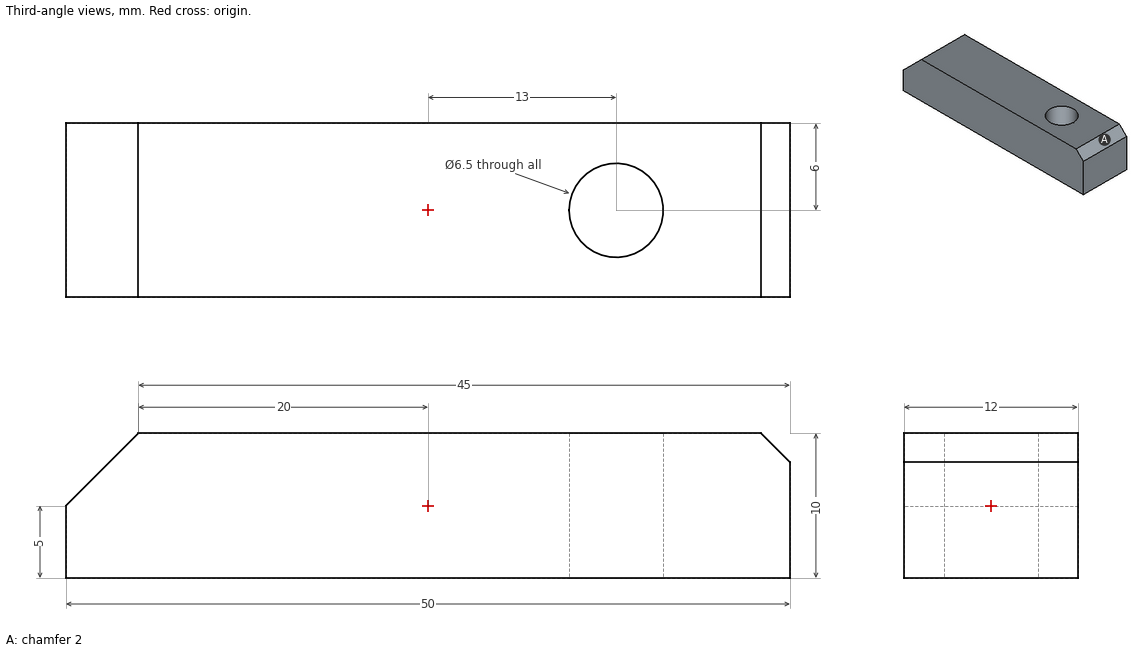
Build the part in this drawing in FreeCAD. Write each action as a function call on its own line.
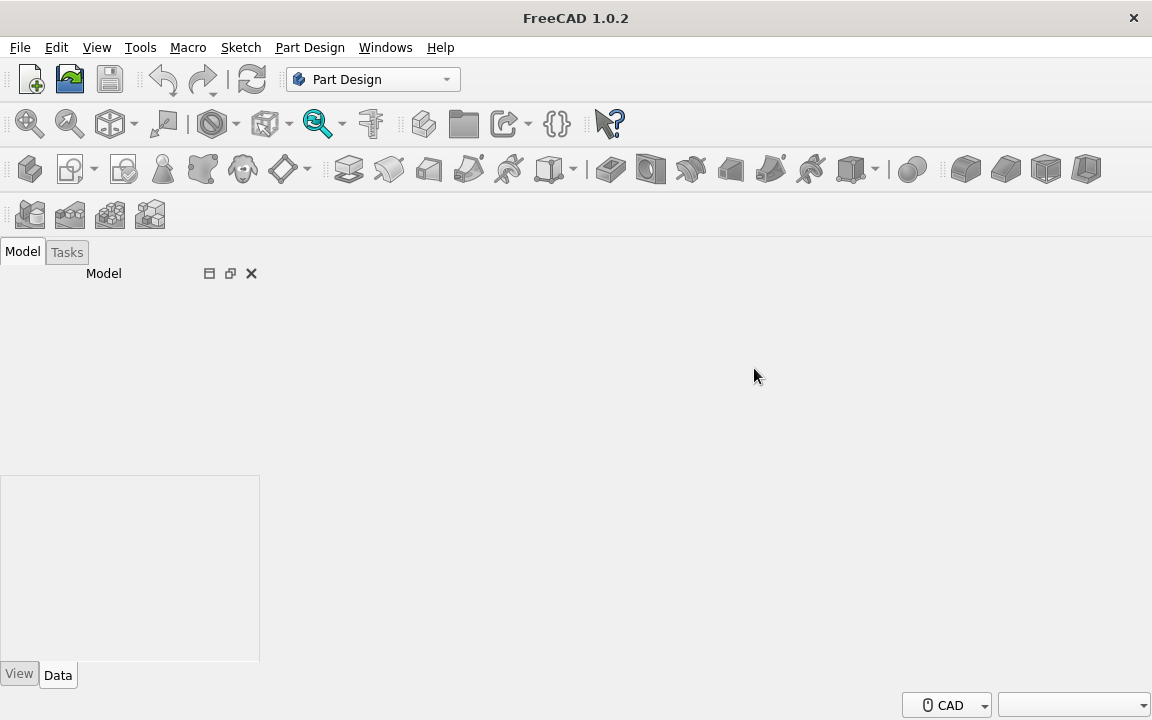
click(30, 80)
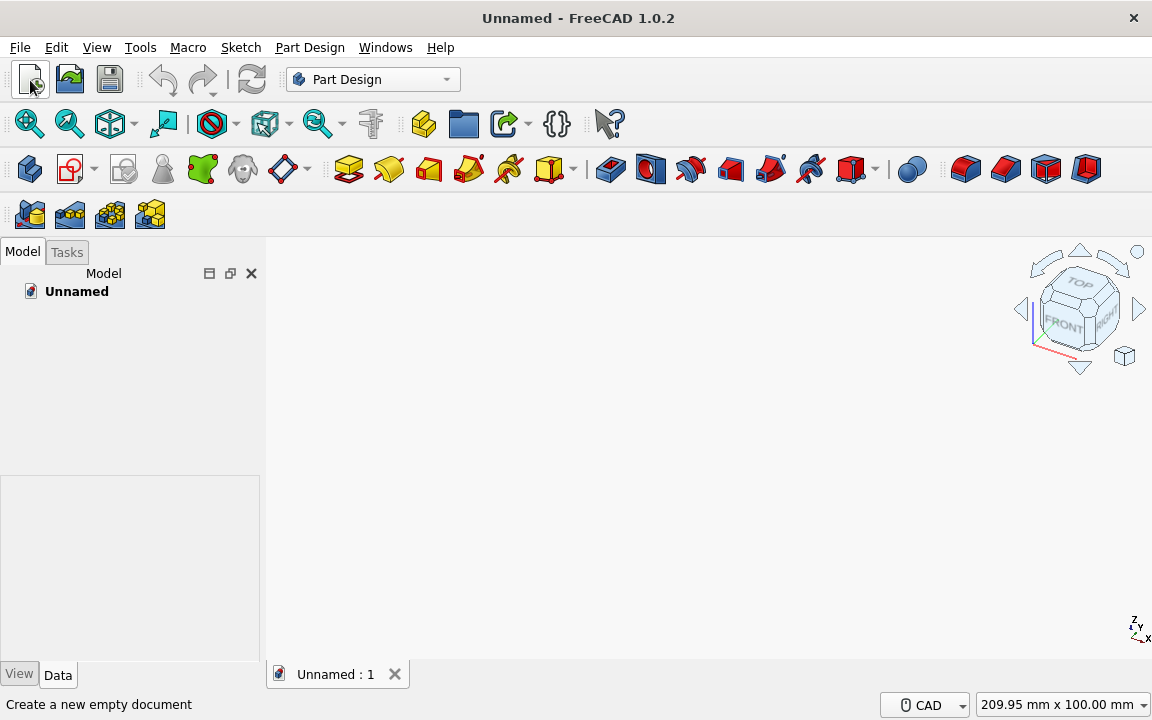
click(30, 170)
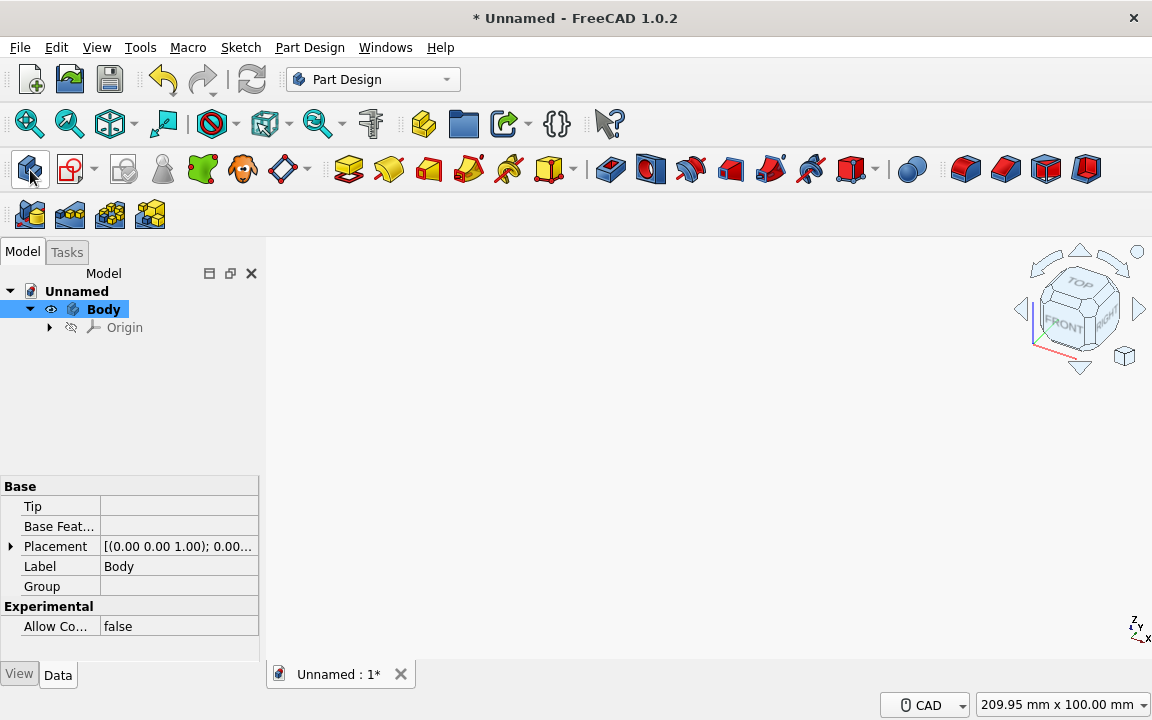
click(50, 327)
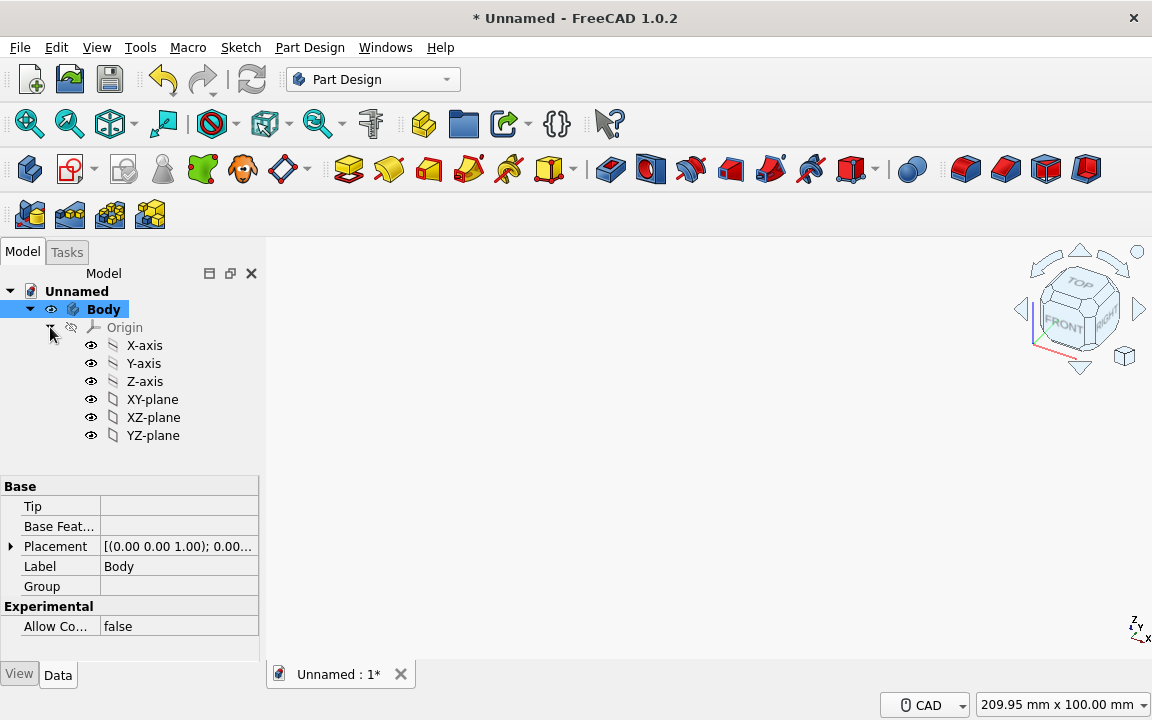
click(136, 417)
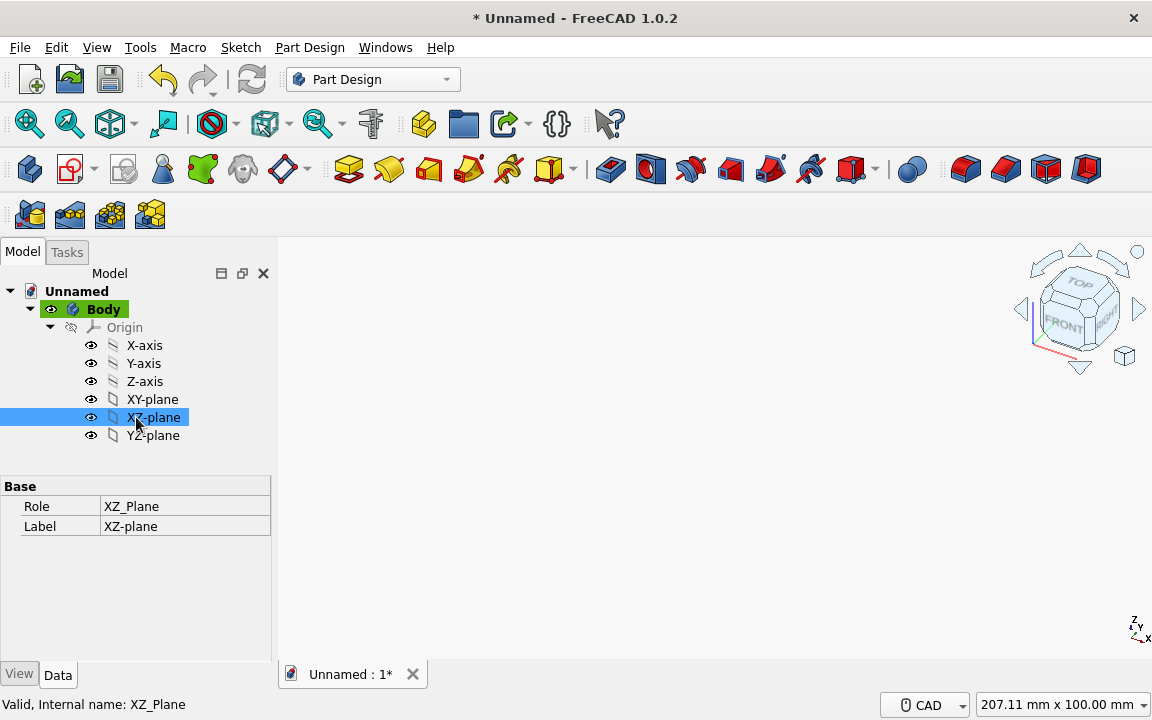
click(284, 170)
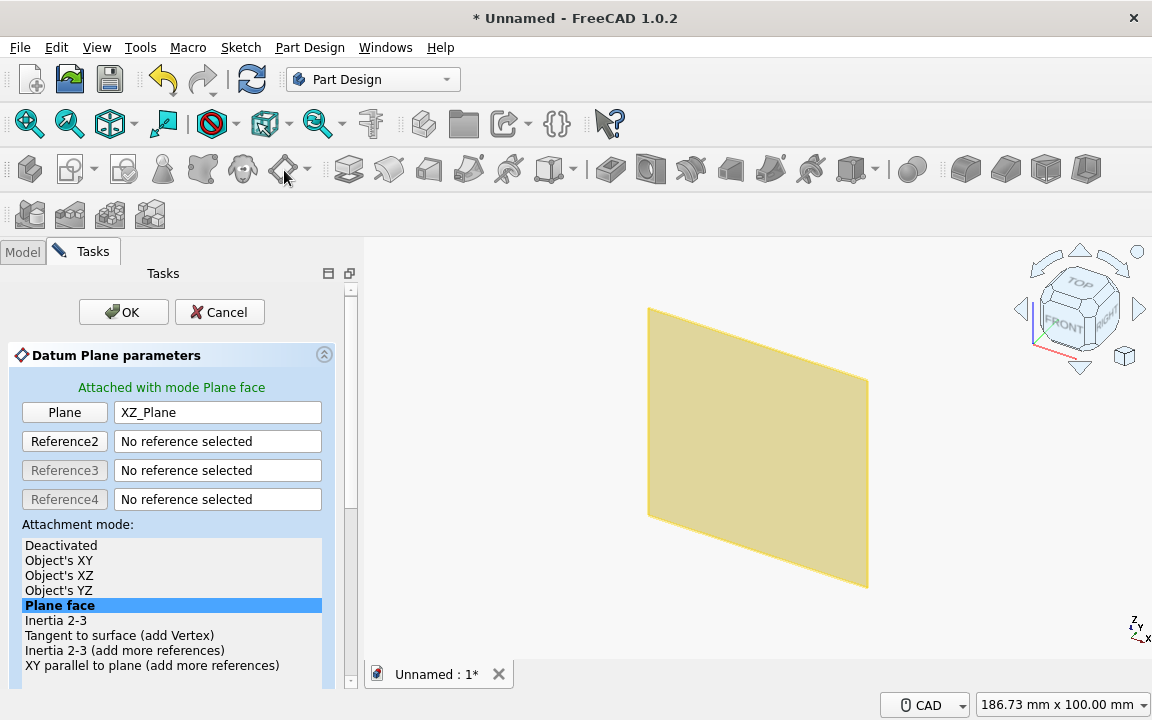
scroll(351, 486, down, 4)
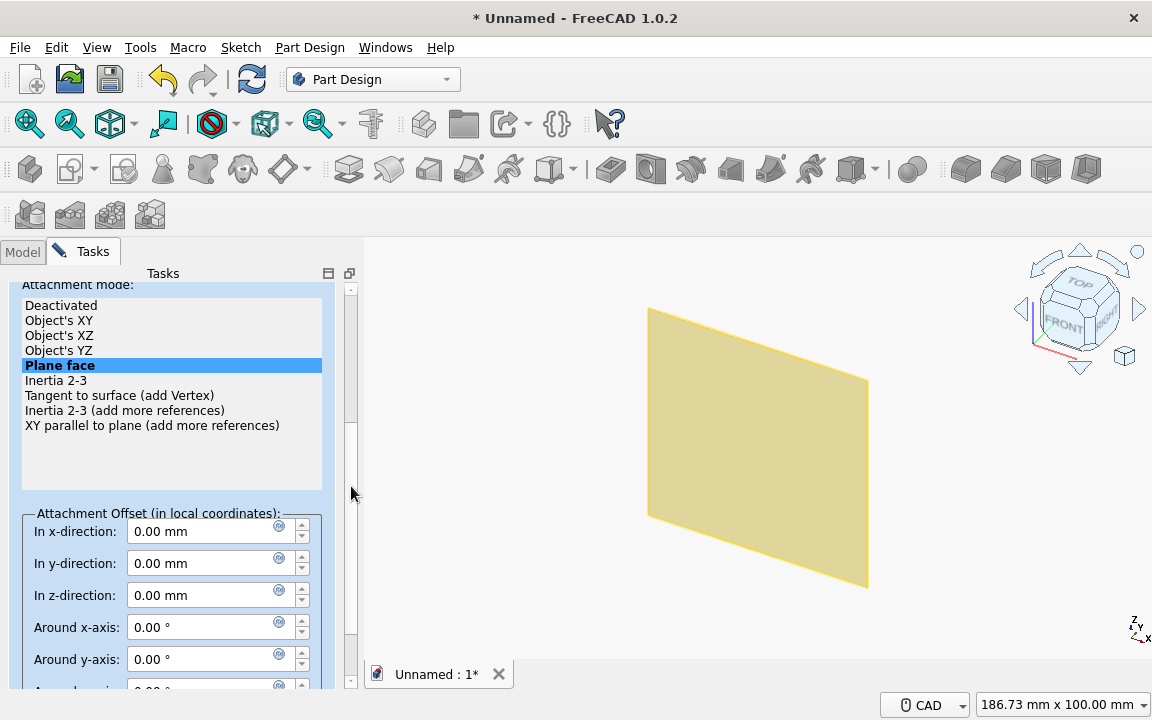
triple_click(210, 595)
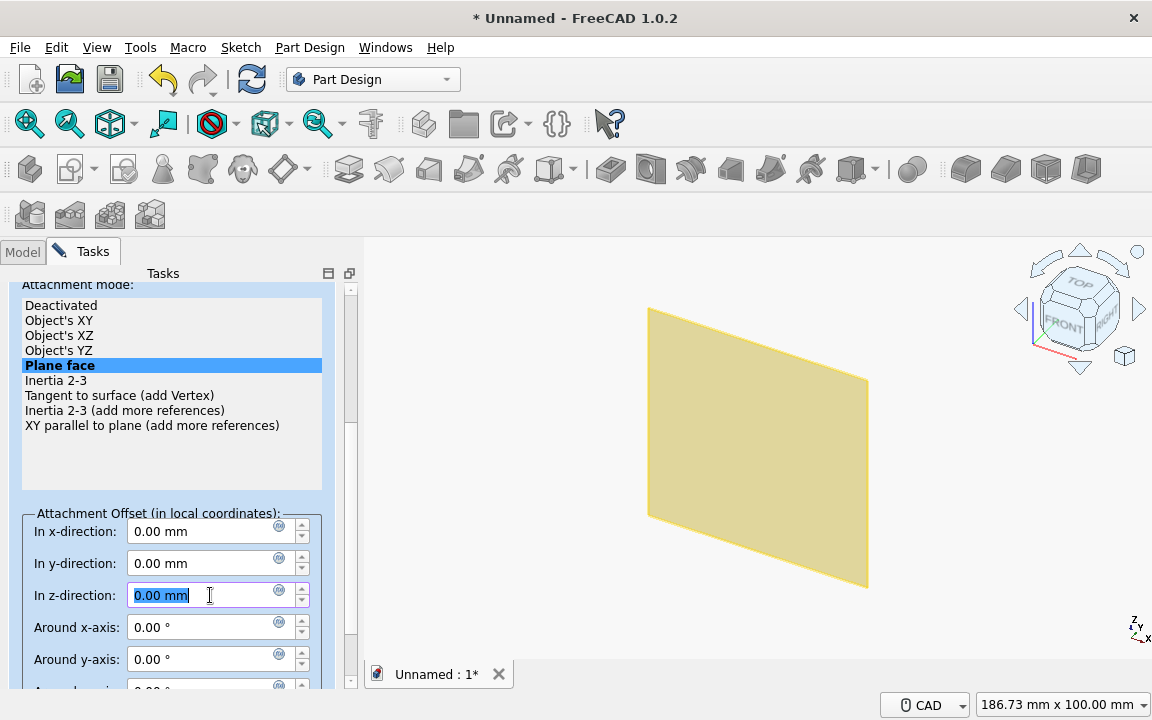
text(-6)
key(Tab)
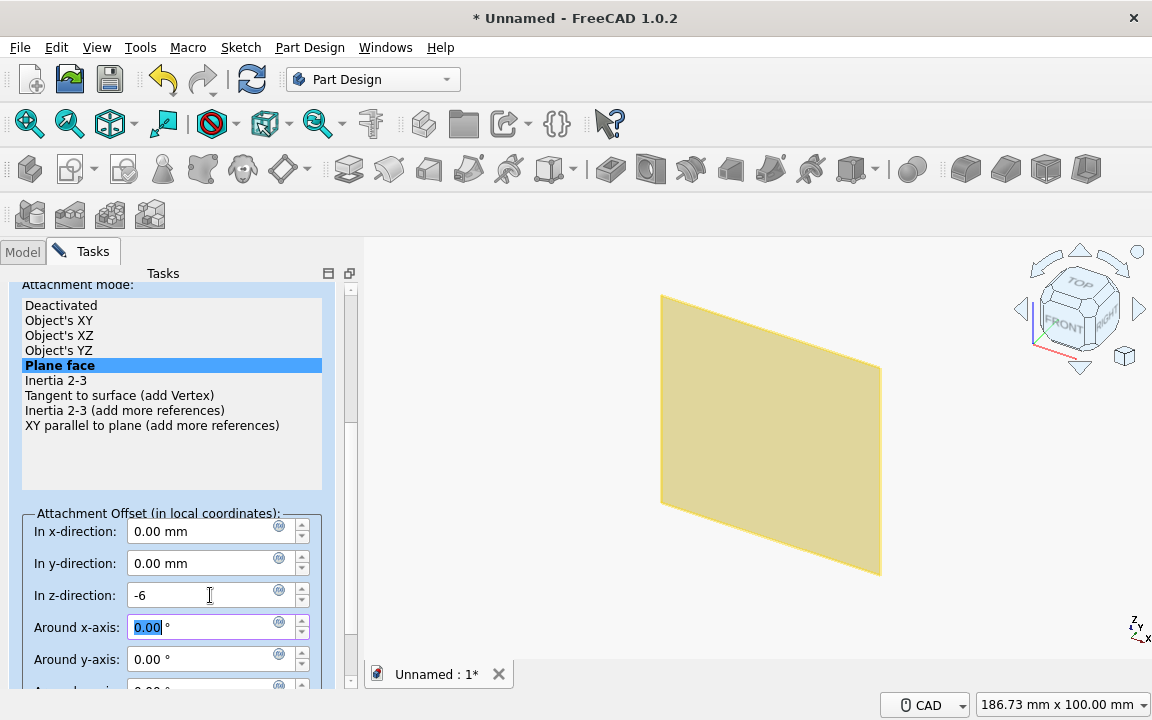
scroll(351, 486, up, 5)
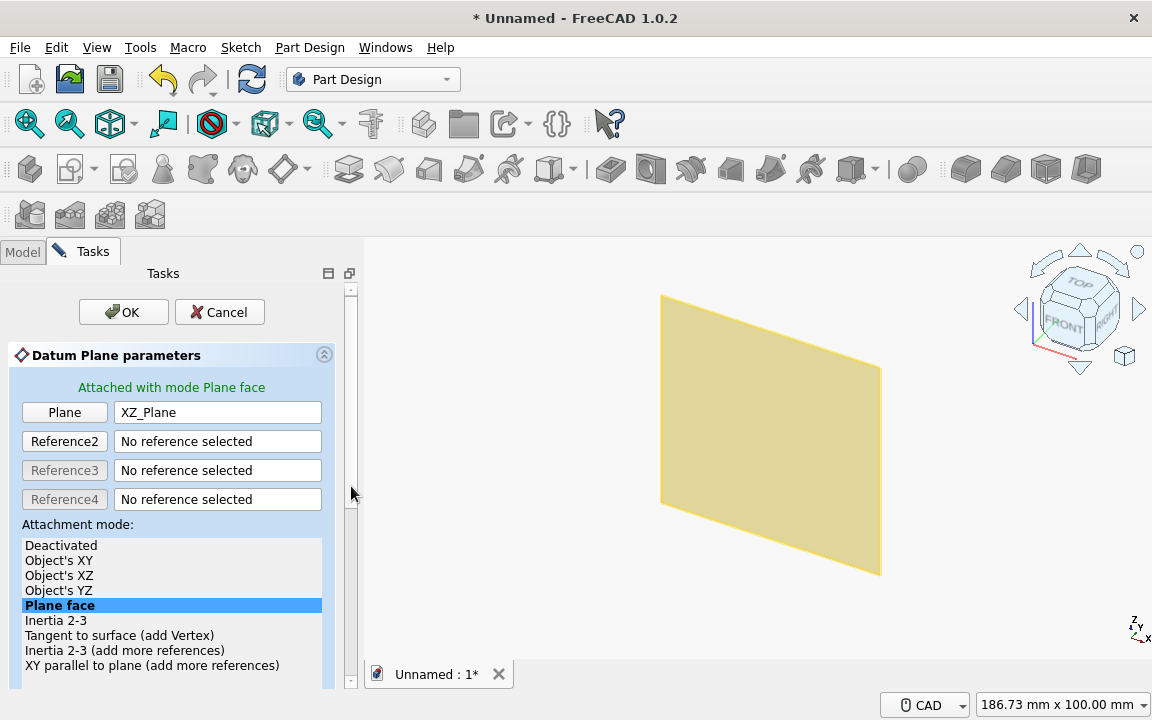
click(124, 312)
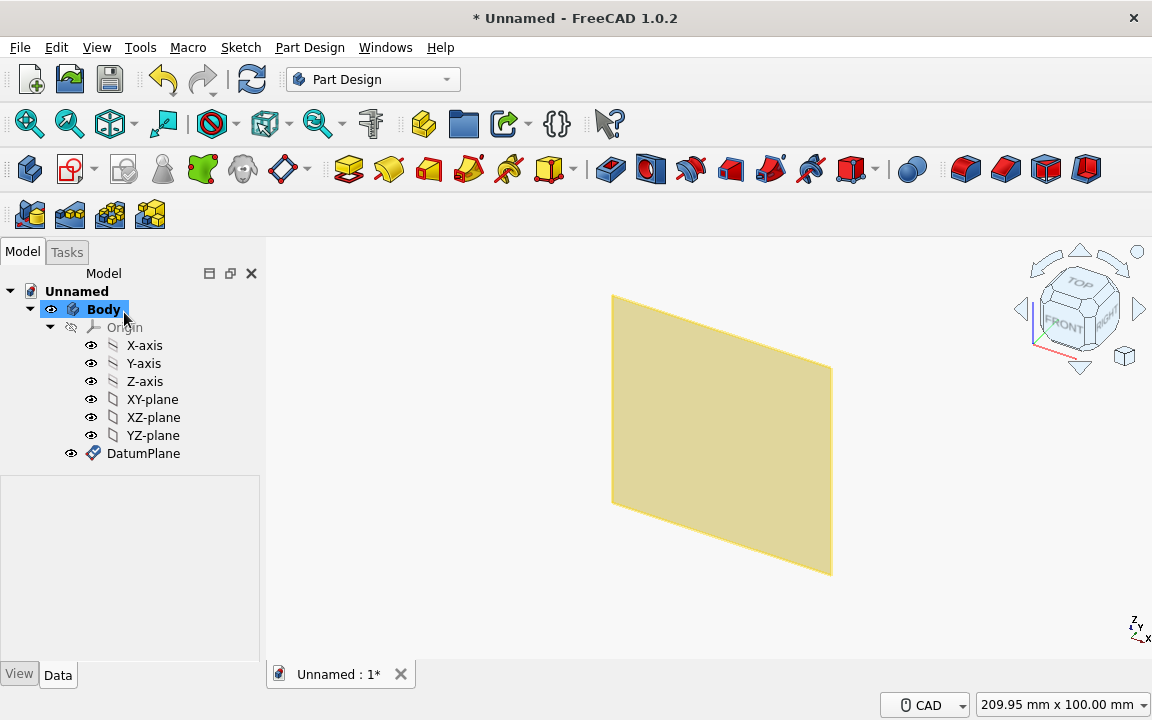
click(116, 453)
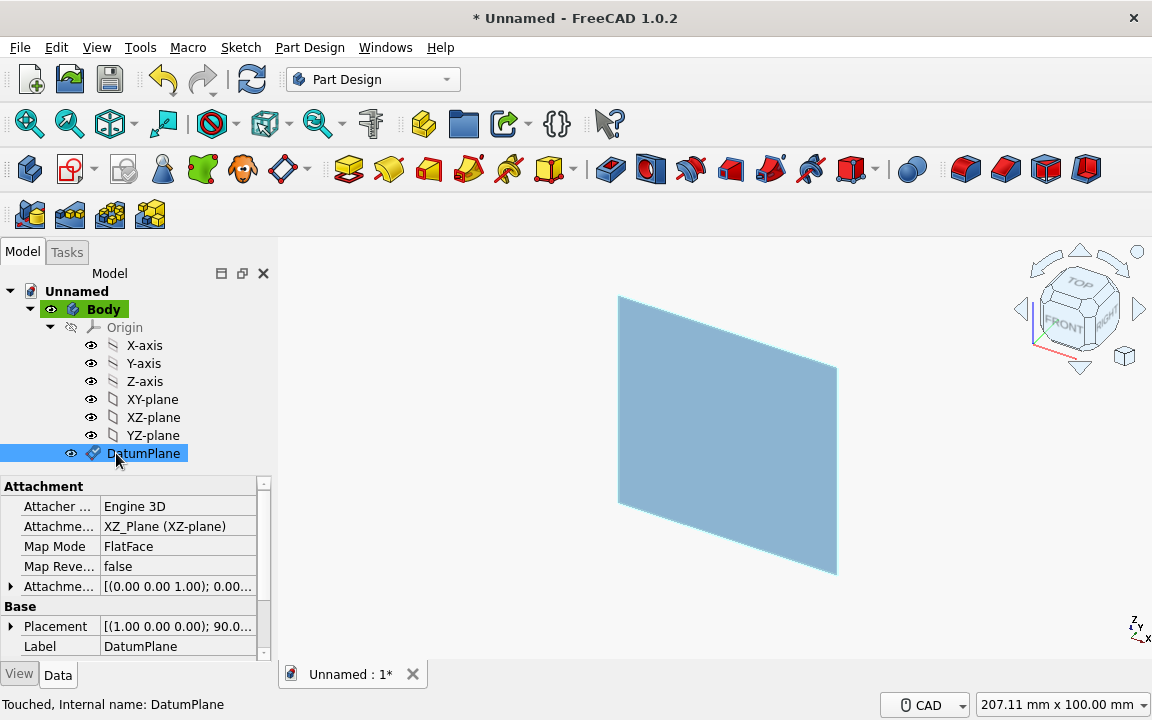
click(70, 170)